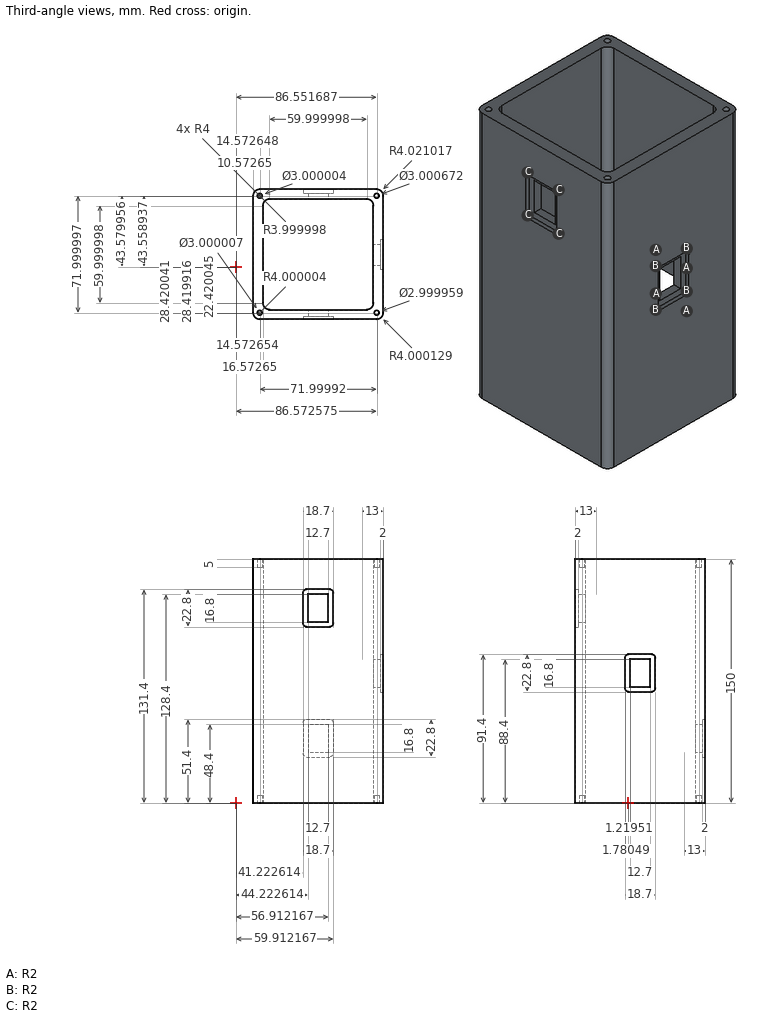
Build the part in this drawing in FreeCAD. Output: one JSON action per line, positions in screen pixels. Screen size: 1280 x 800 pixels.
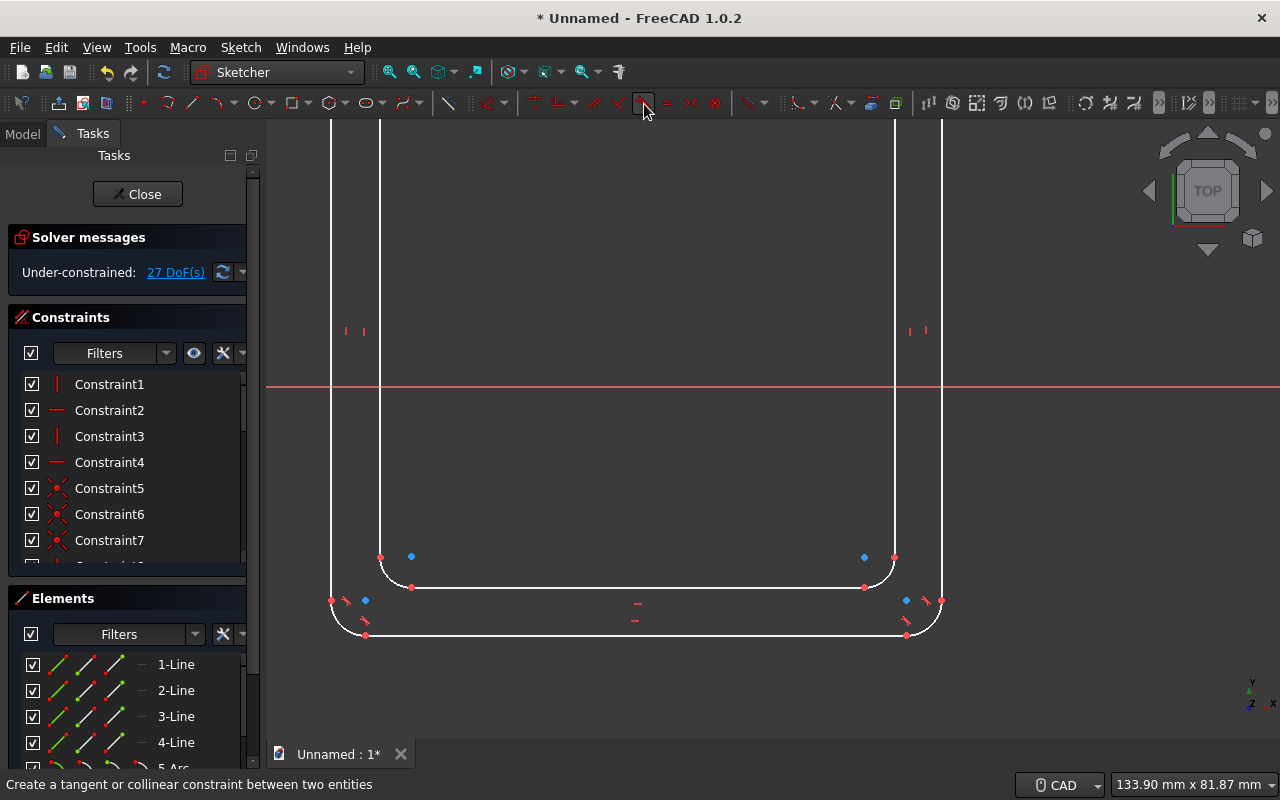
{"action": "left_click", "coordinate": [942, 438]}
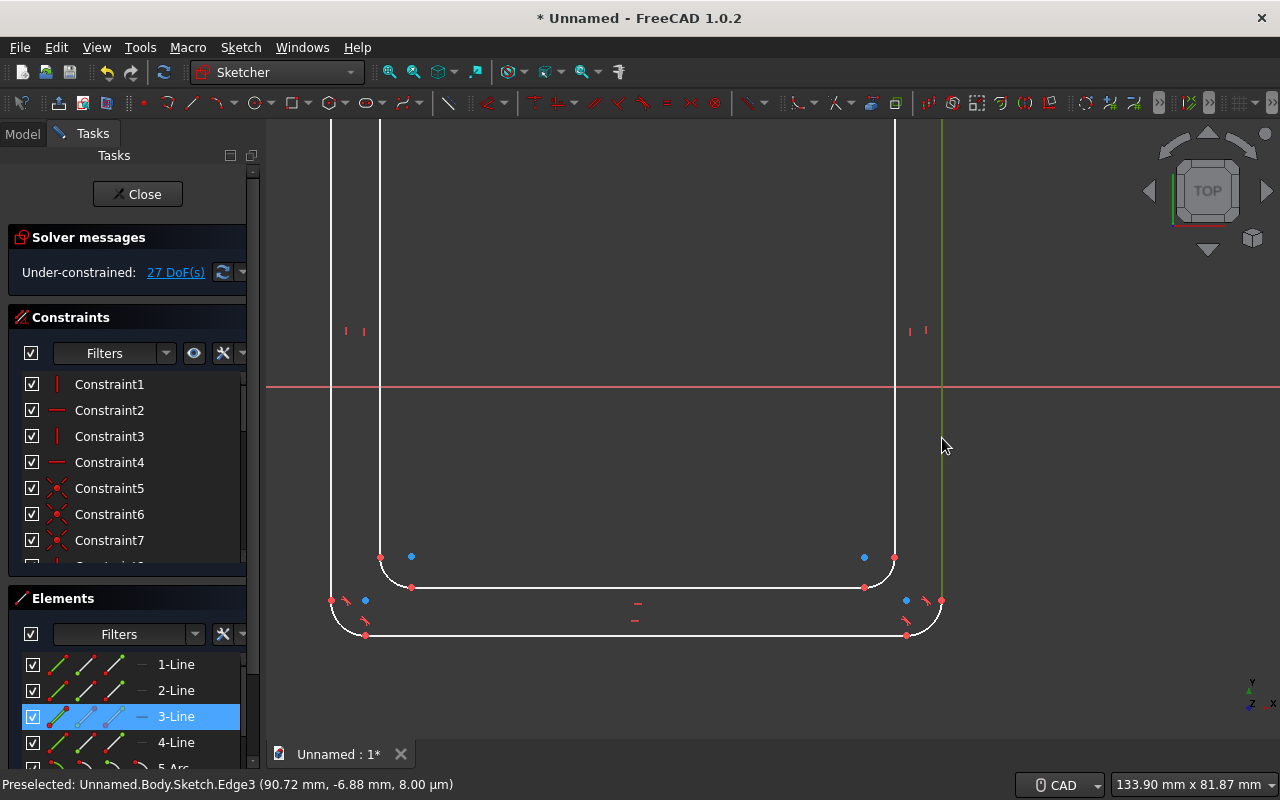
{"action": "scroll", "coordinate": [921, 631], "scroll_direction": "down", "scroll_amount": 2}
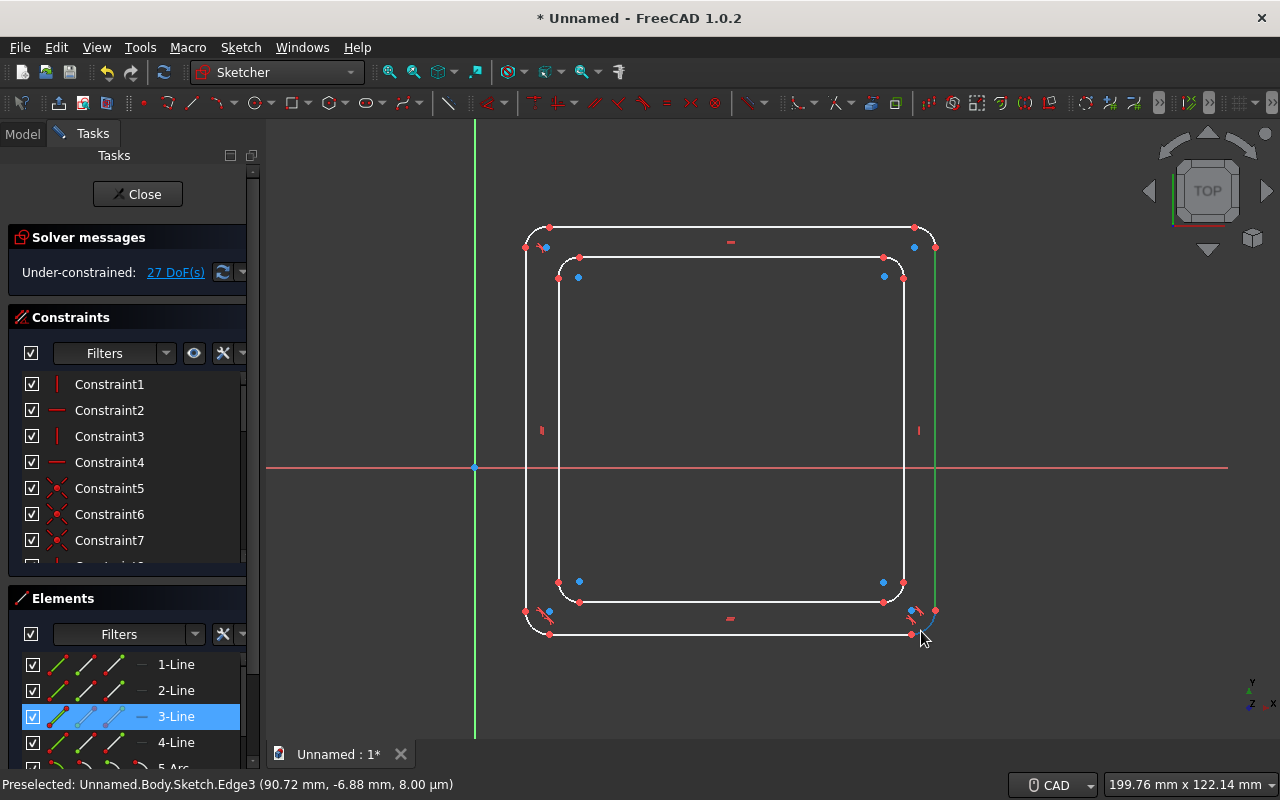
{"action": "scroll", "coordinate": [933, 238], "scroll_direction": "up", "scroll_amount": 2}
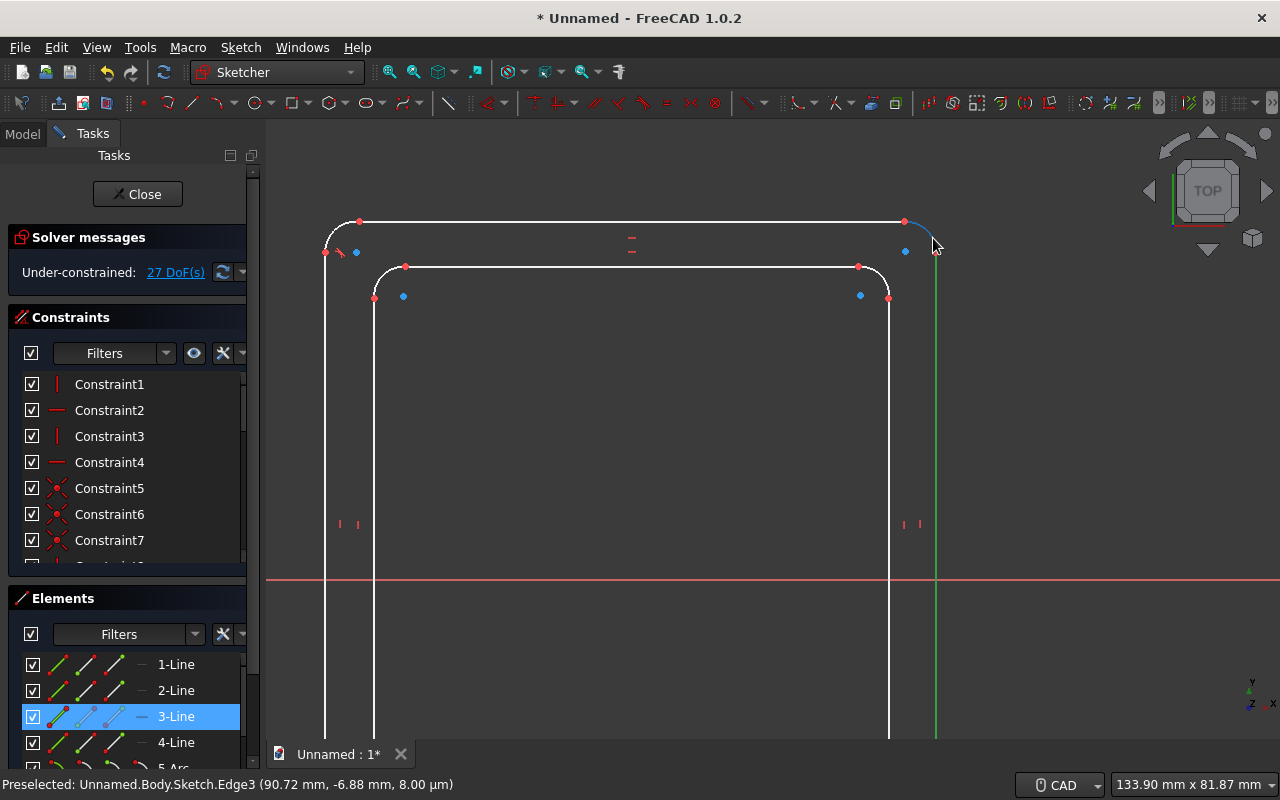
{"action": "left_click", "coordinate": [933, 238]}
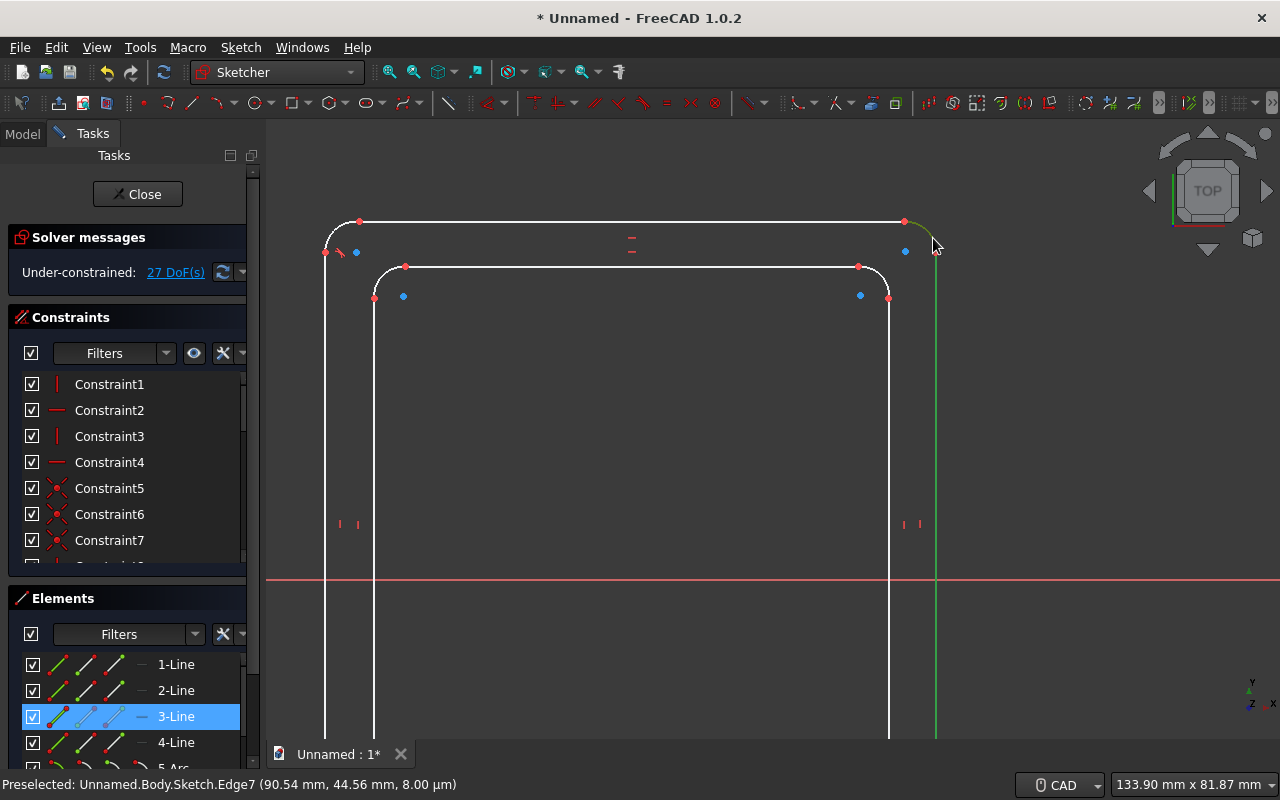
{"action": "left_click", "coordinate": [644, 104]}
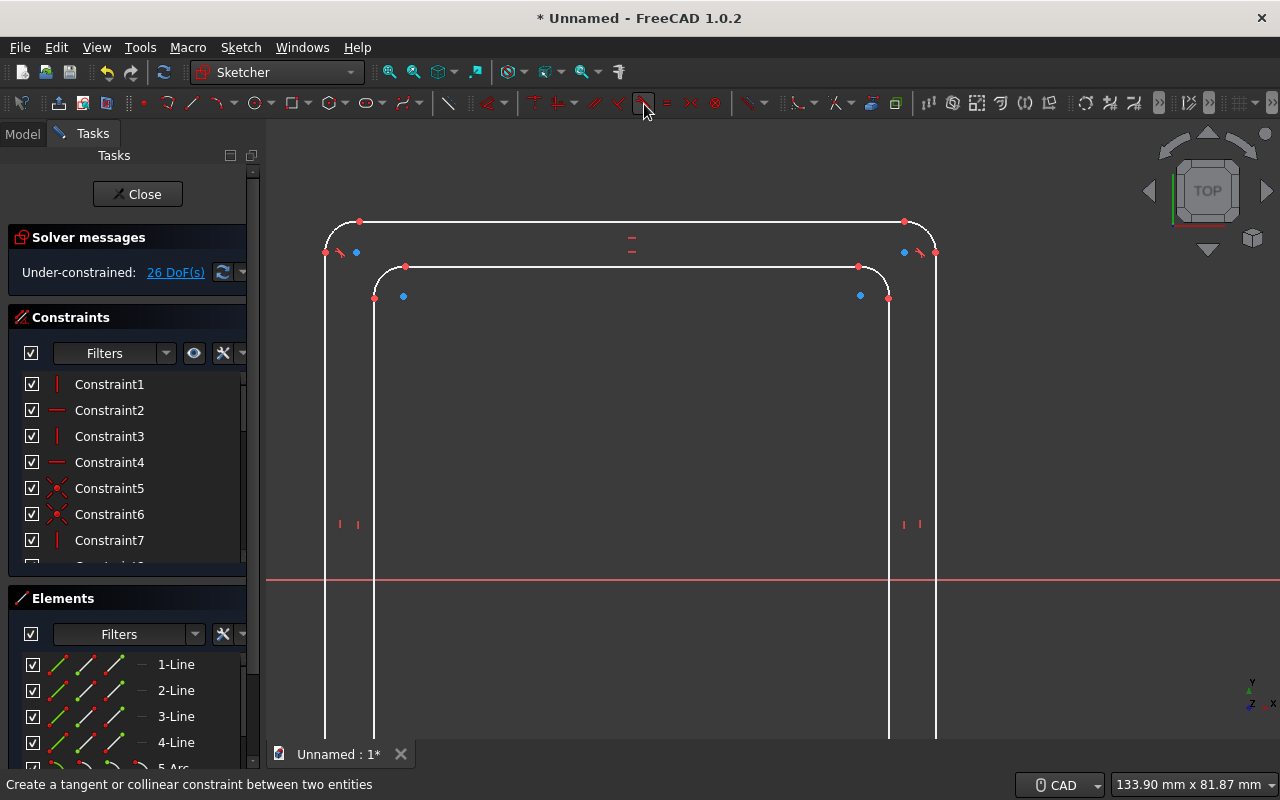
{"action": "left_click", "coordinate": [741, 222]}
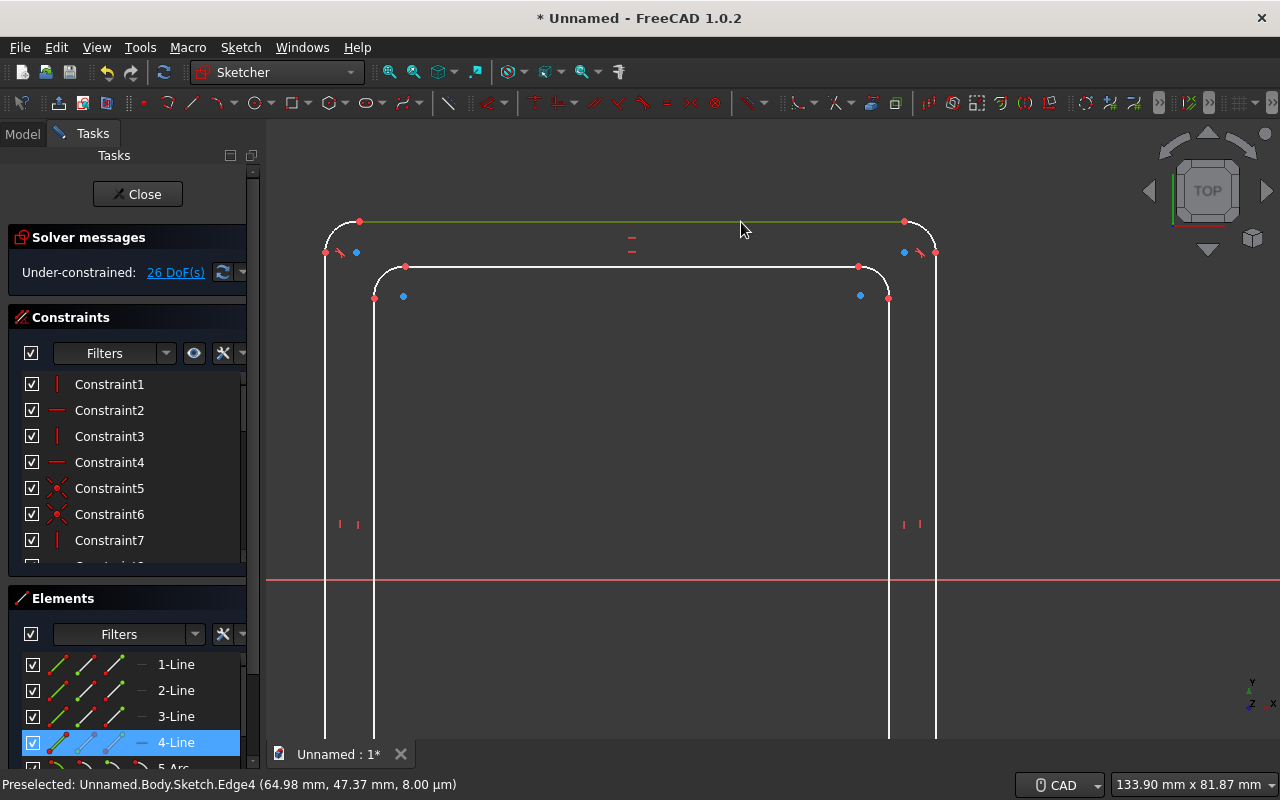
{"action": "left_click", "coordinate": [933, 239]}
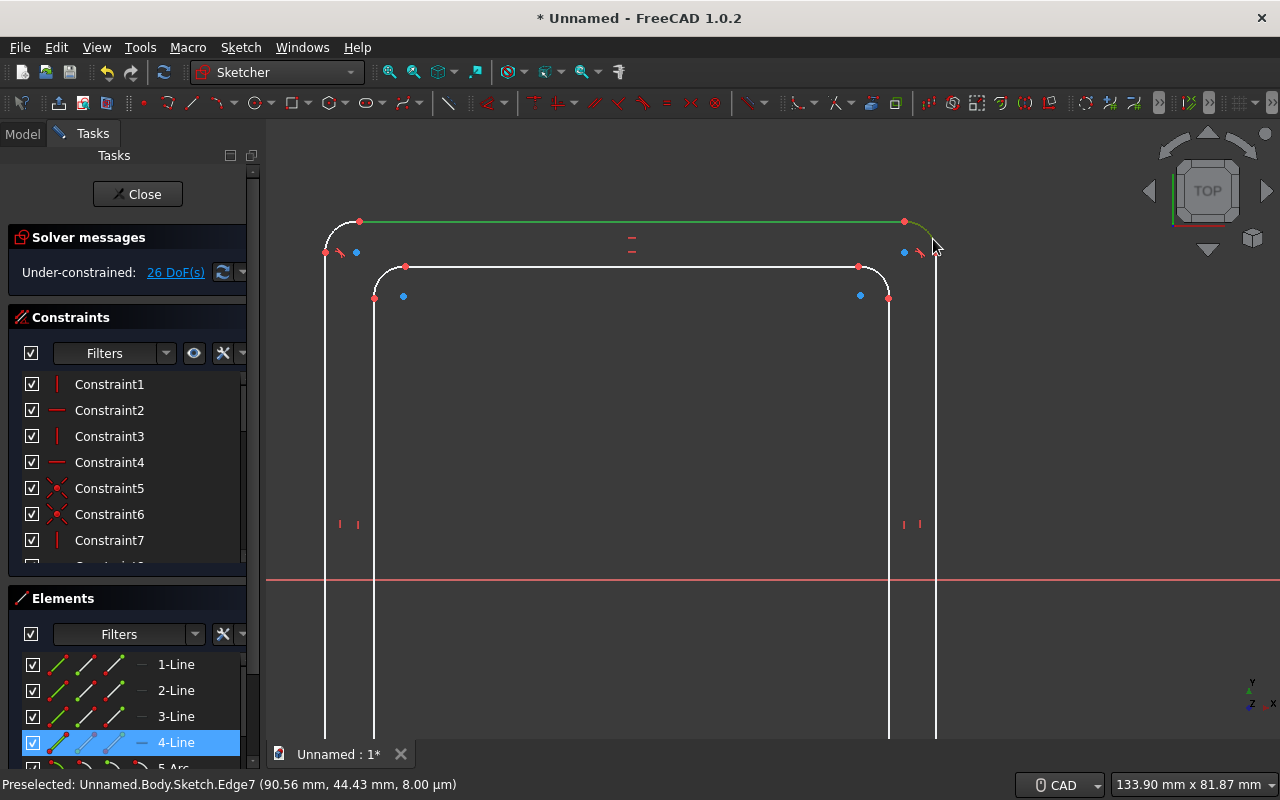
{"action": "left_click", "coordinate": [644, 104]}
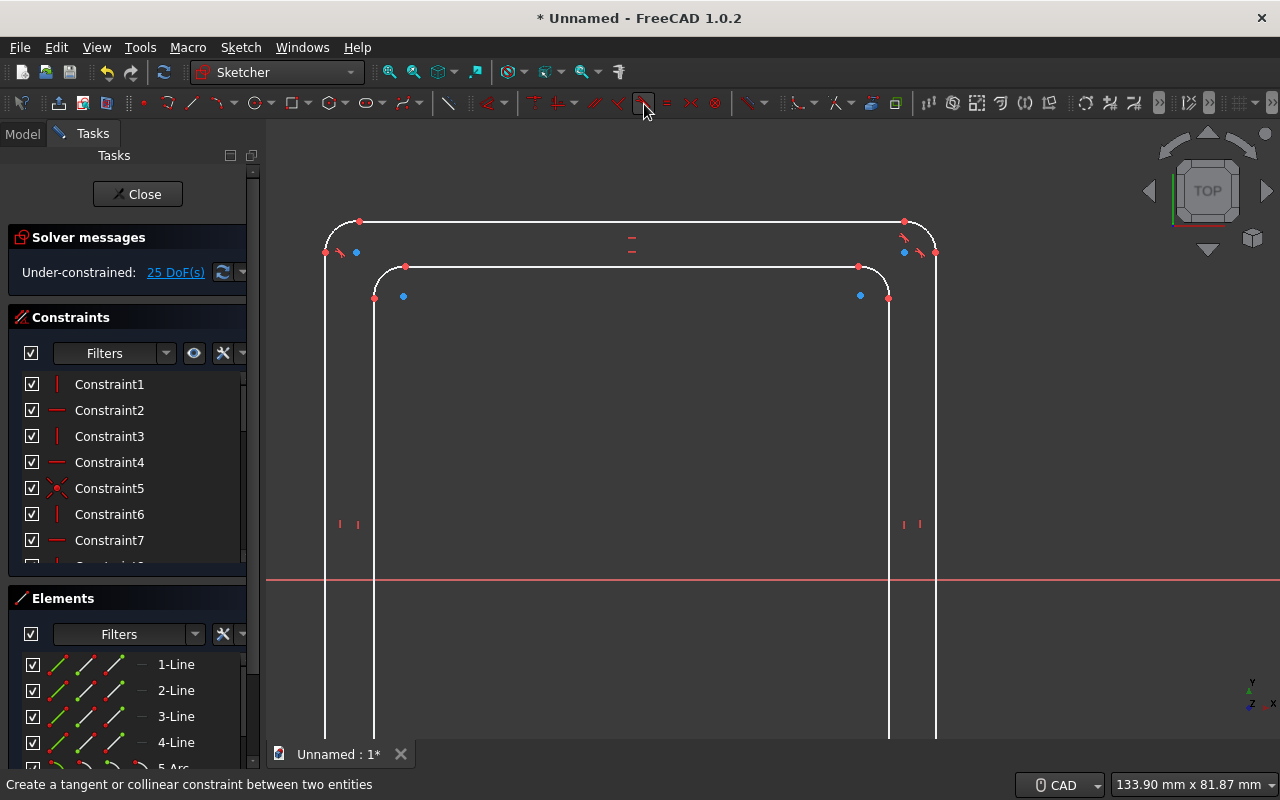
{"action": "left_click", "coordinate": [741, 222]}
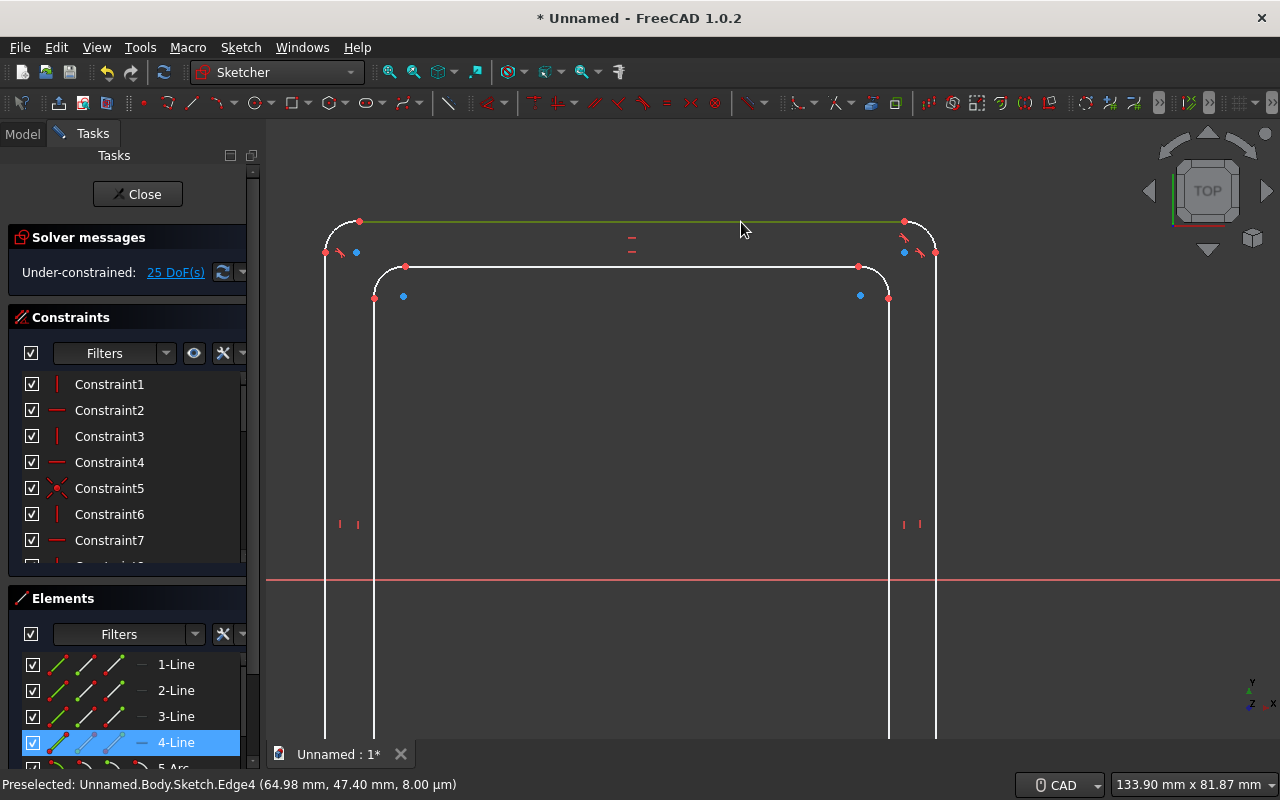
{"action": "left_click", "coordinate": [344, 224]}